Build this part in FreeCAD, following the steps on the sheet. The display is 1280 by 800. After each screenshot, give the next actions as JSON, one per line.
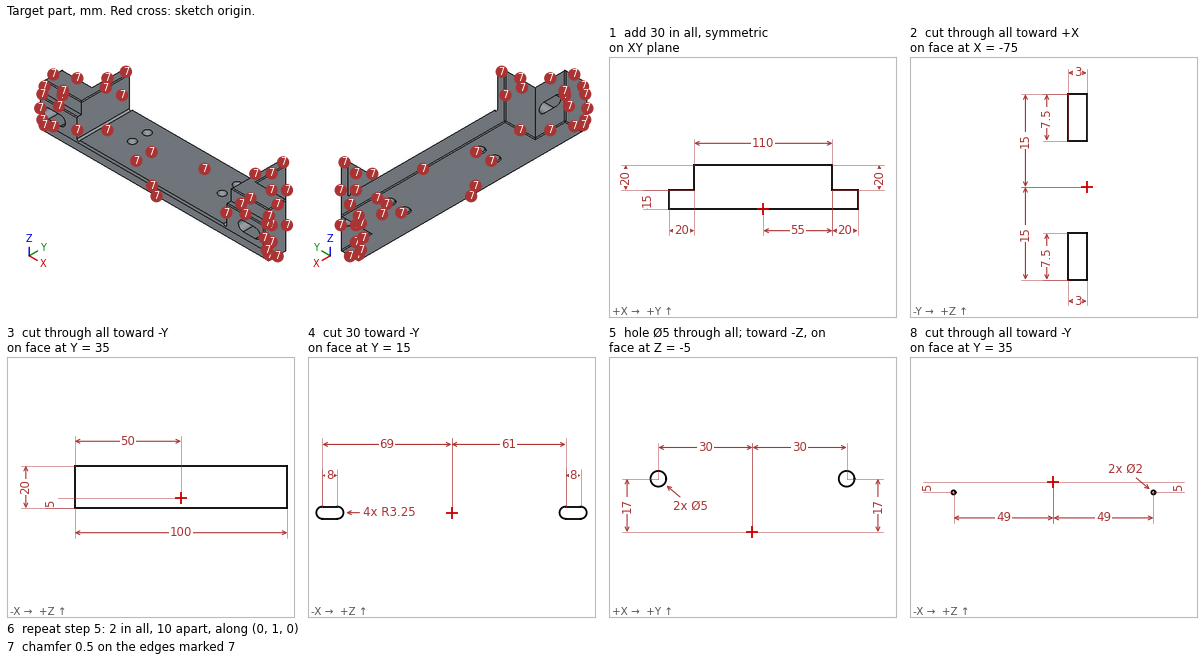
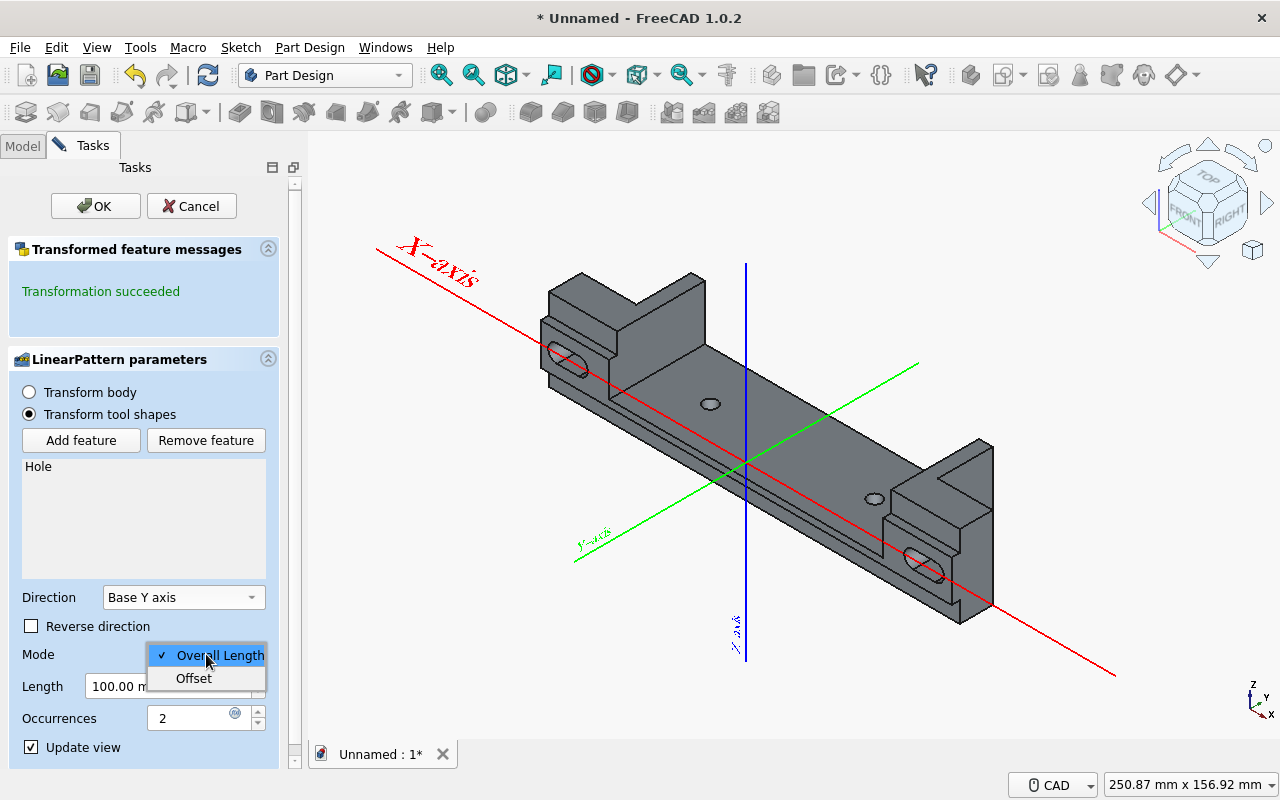
{"action": "left_click", "coordinate": [206, 678]}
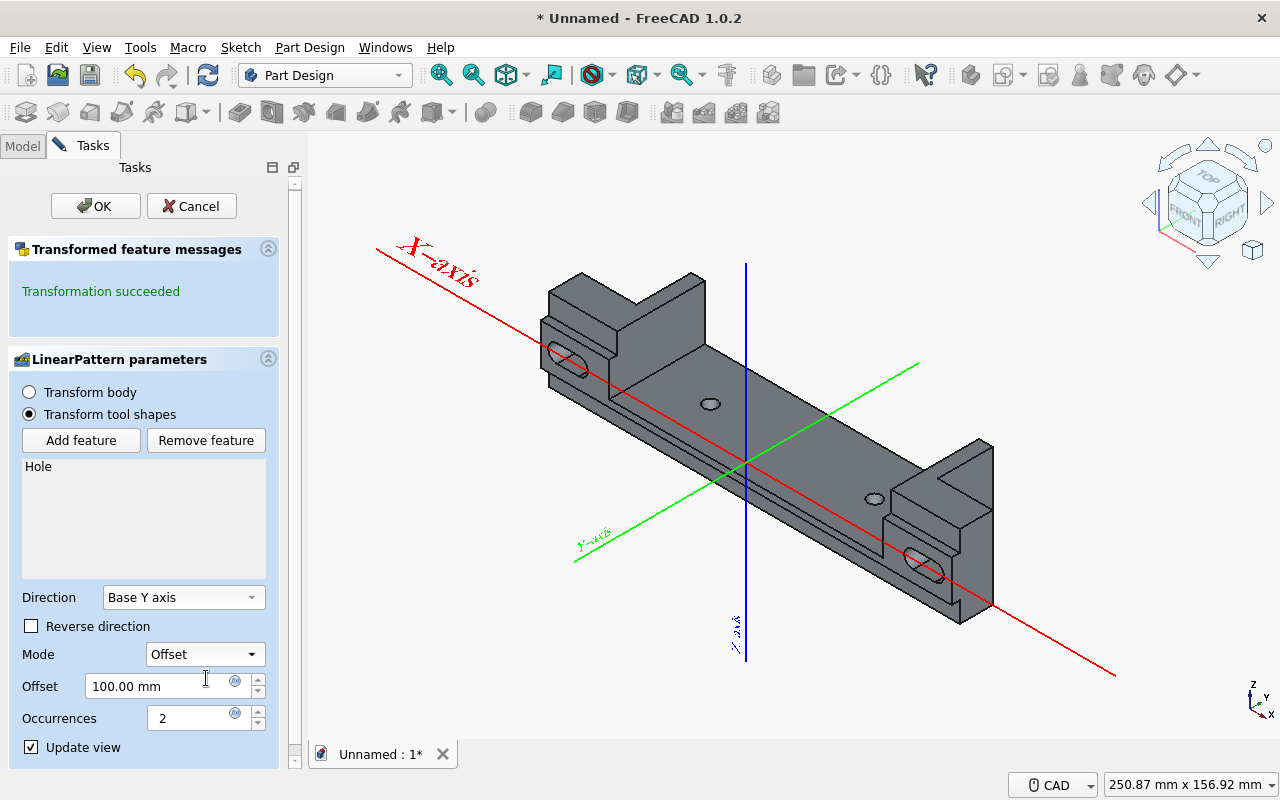
{"action": "triple_click", "coordinate": [168, 686]}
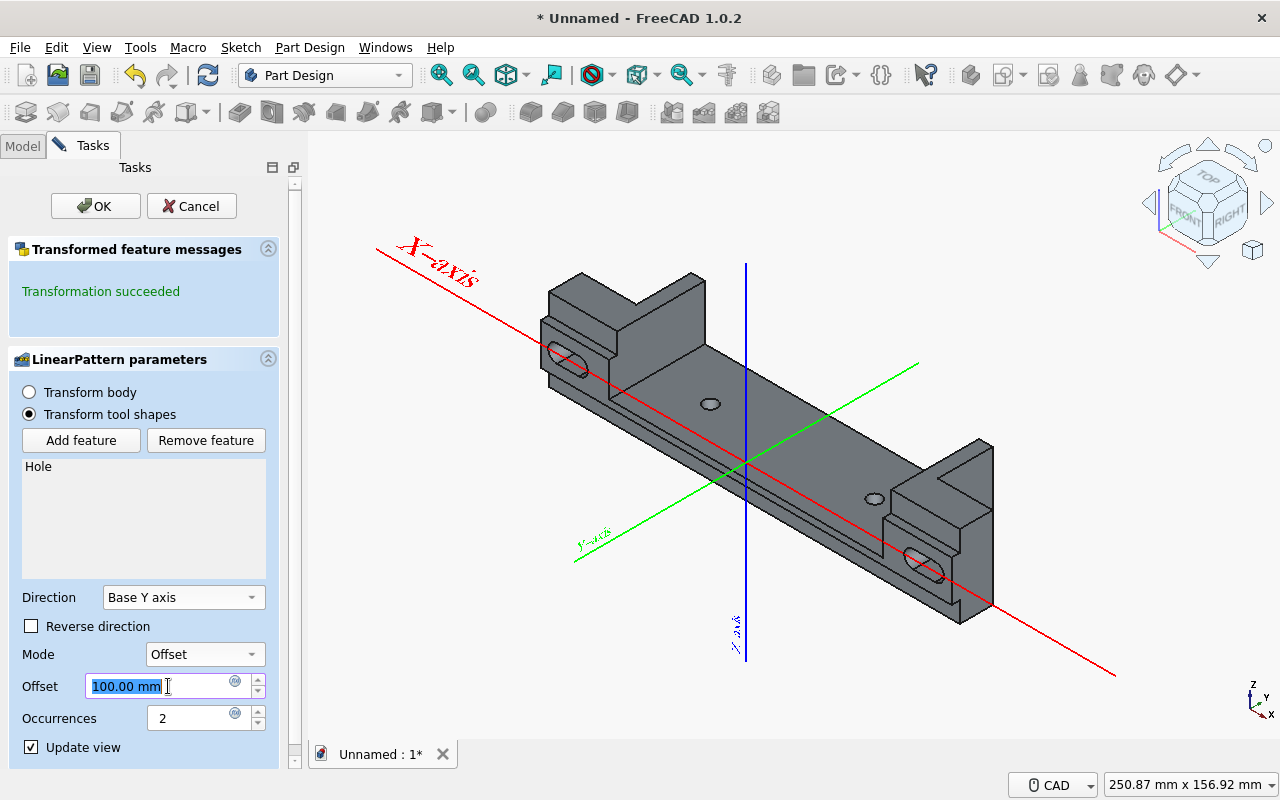
{"action": "type", "text": "10"}
{"action": "key", "text": "Tab"}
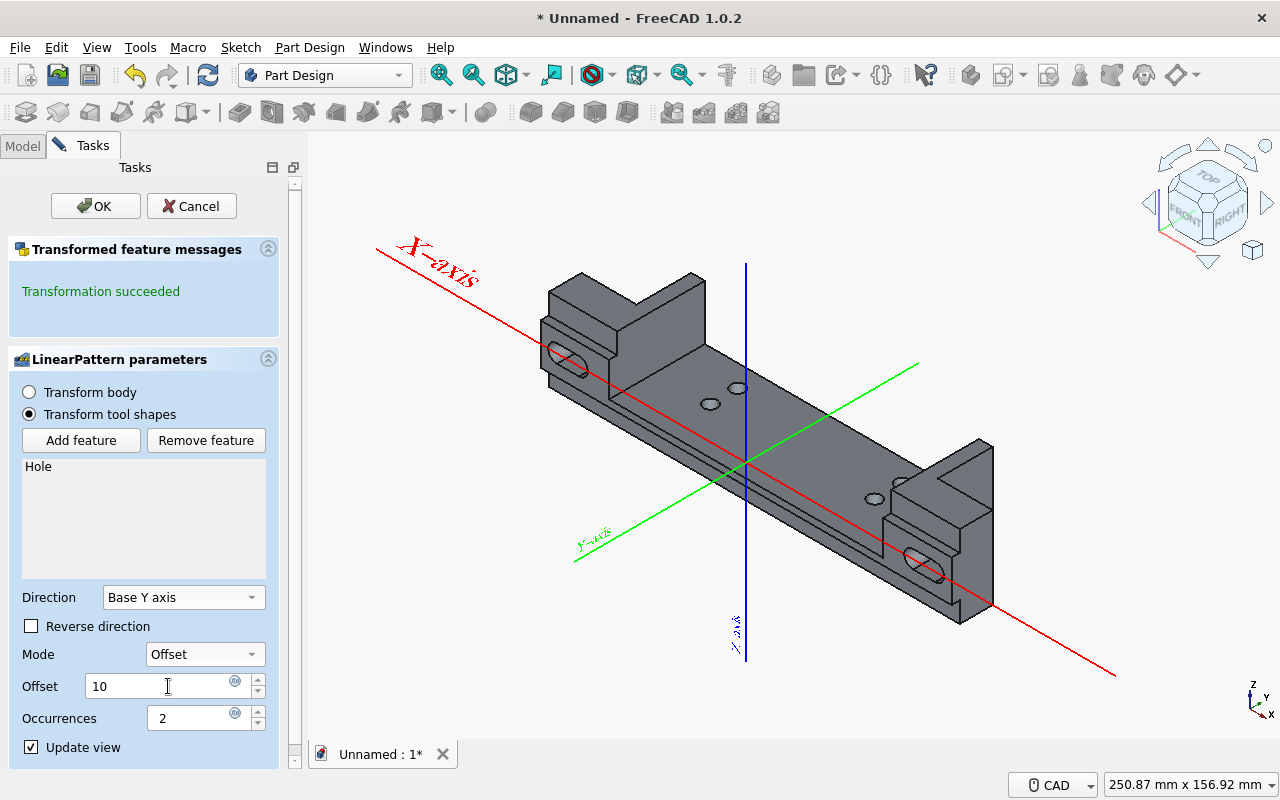
{"action": "triple_click", "coordinate": [198, 718]}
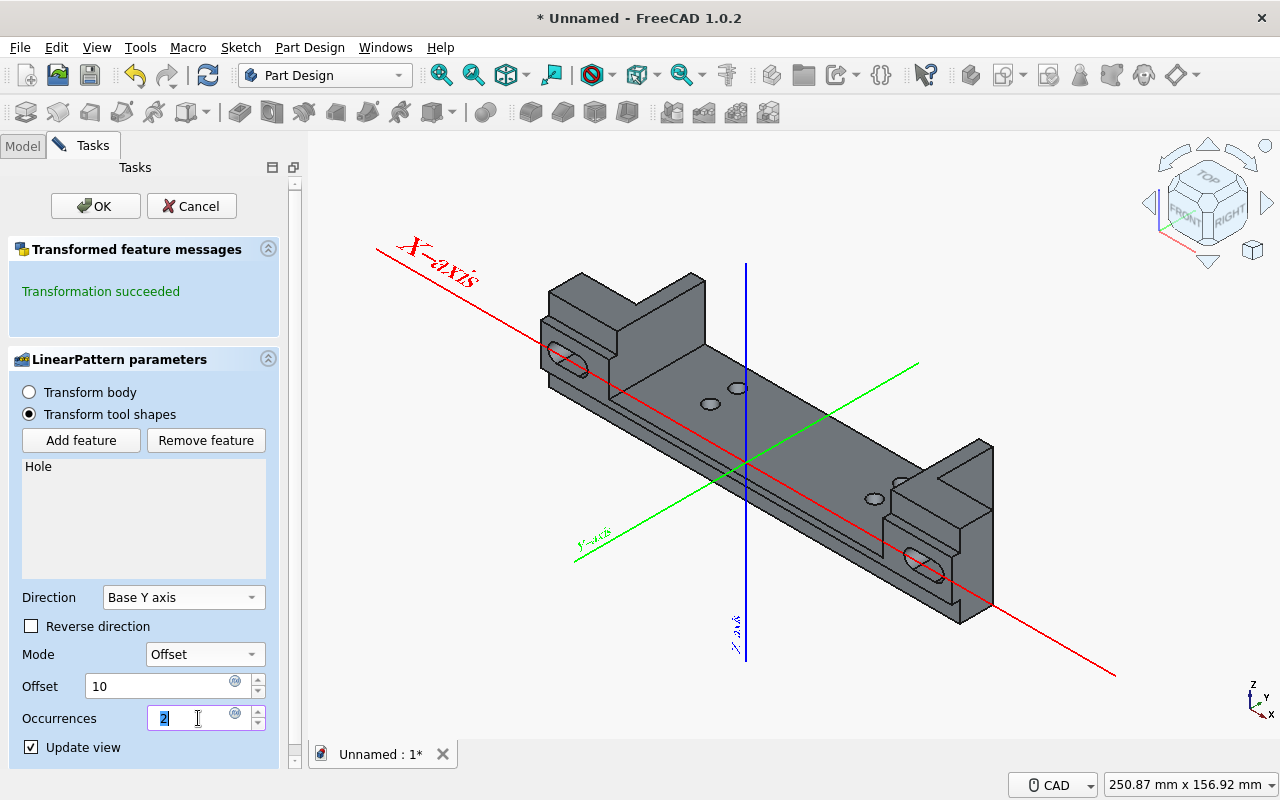
{"action": "type", "text": "2"}
{"action": "key", "text": "Tab"}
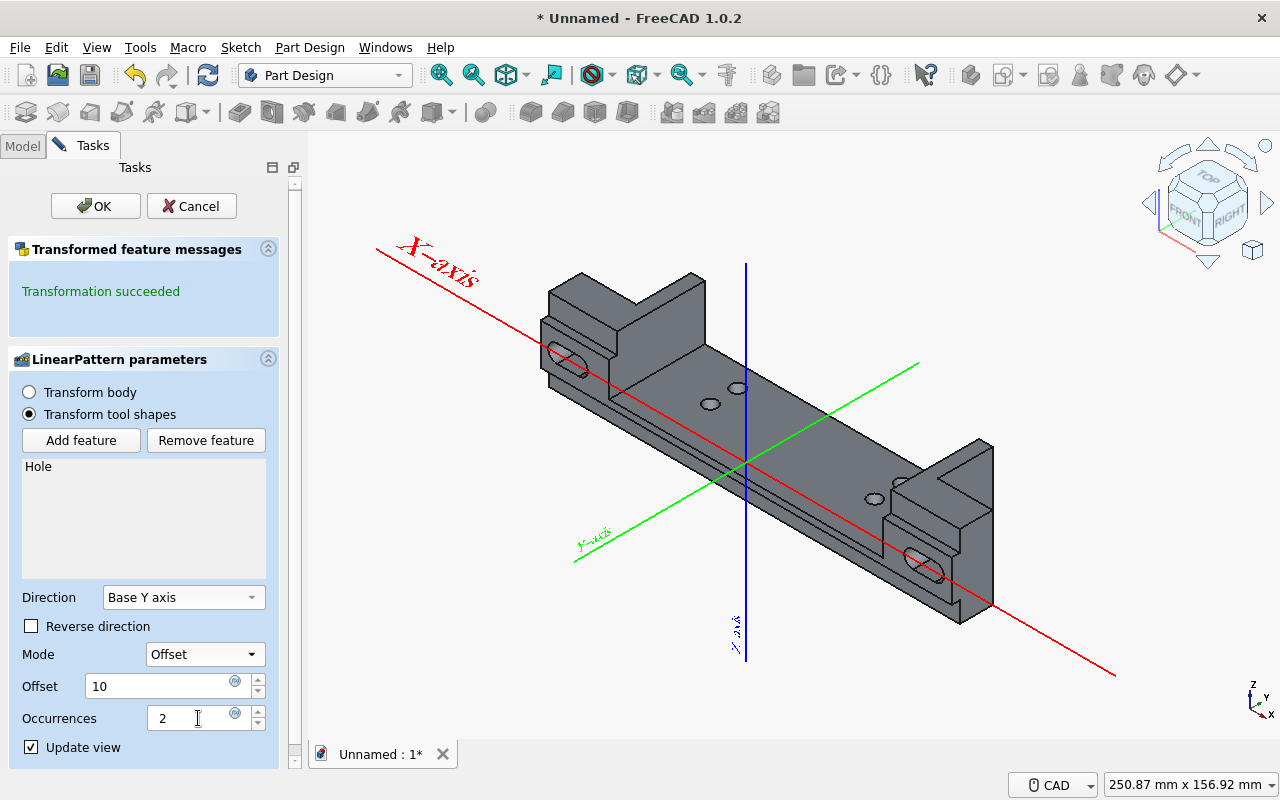
{"action": "left_click", "coordinate": [96, 206]}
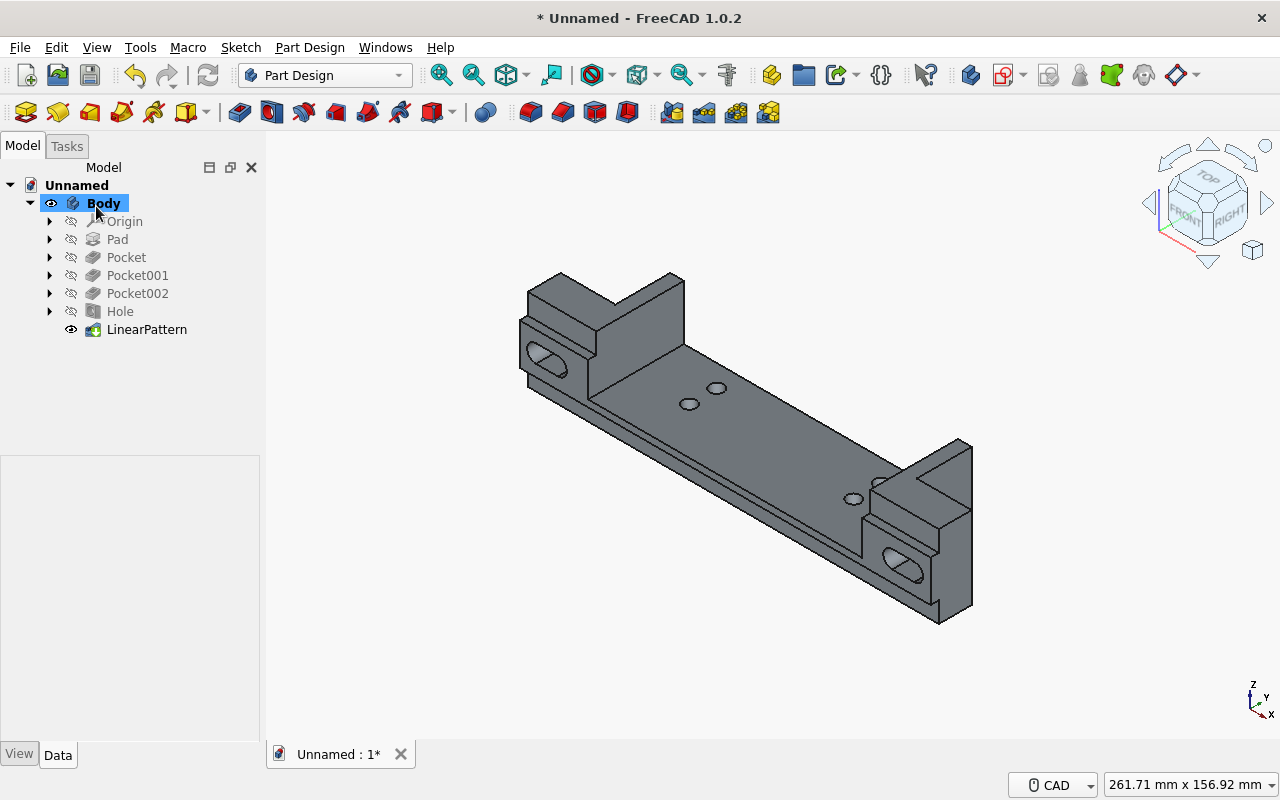
{"action": "left_click", "coordinate": [951, 568]}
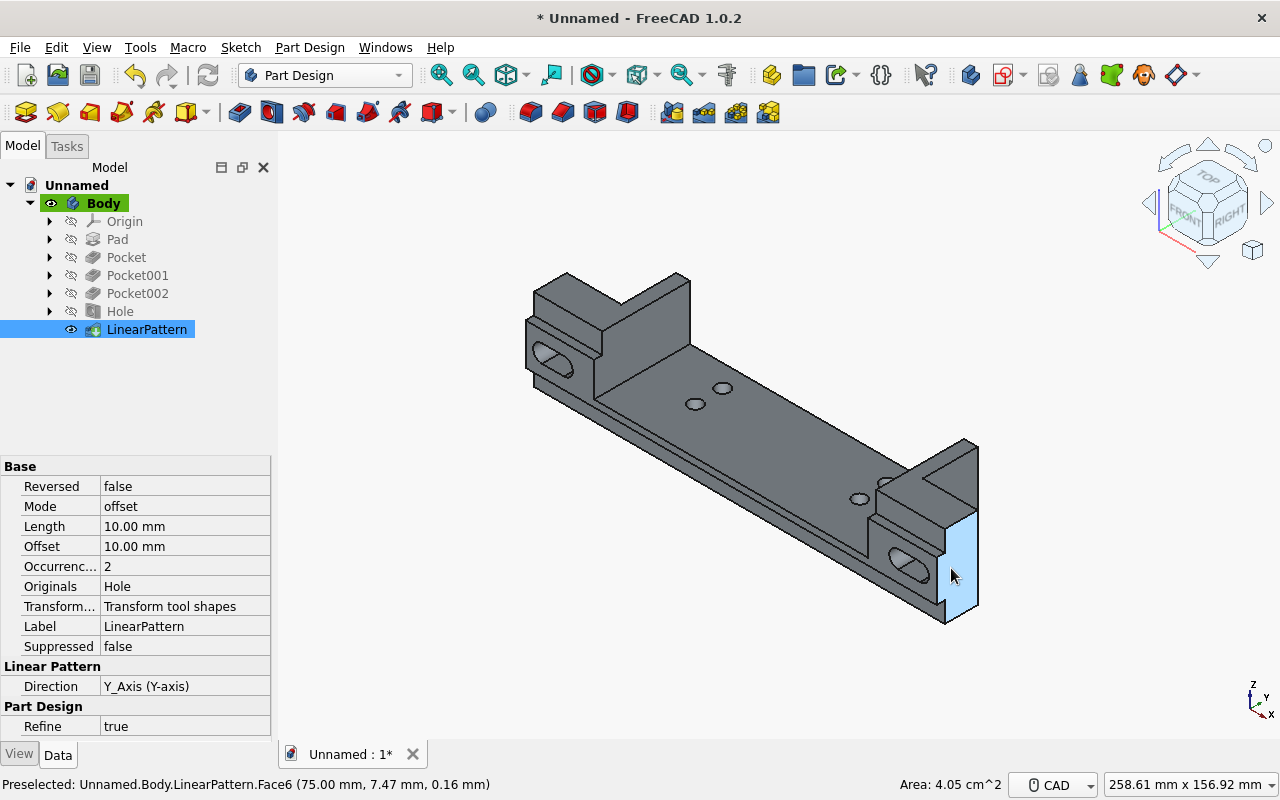
{"action": "left_click", "coordinate": [606, 311], "text": "ctrl"}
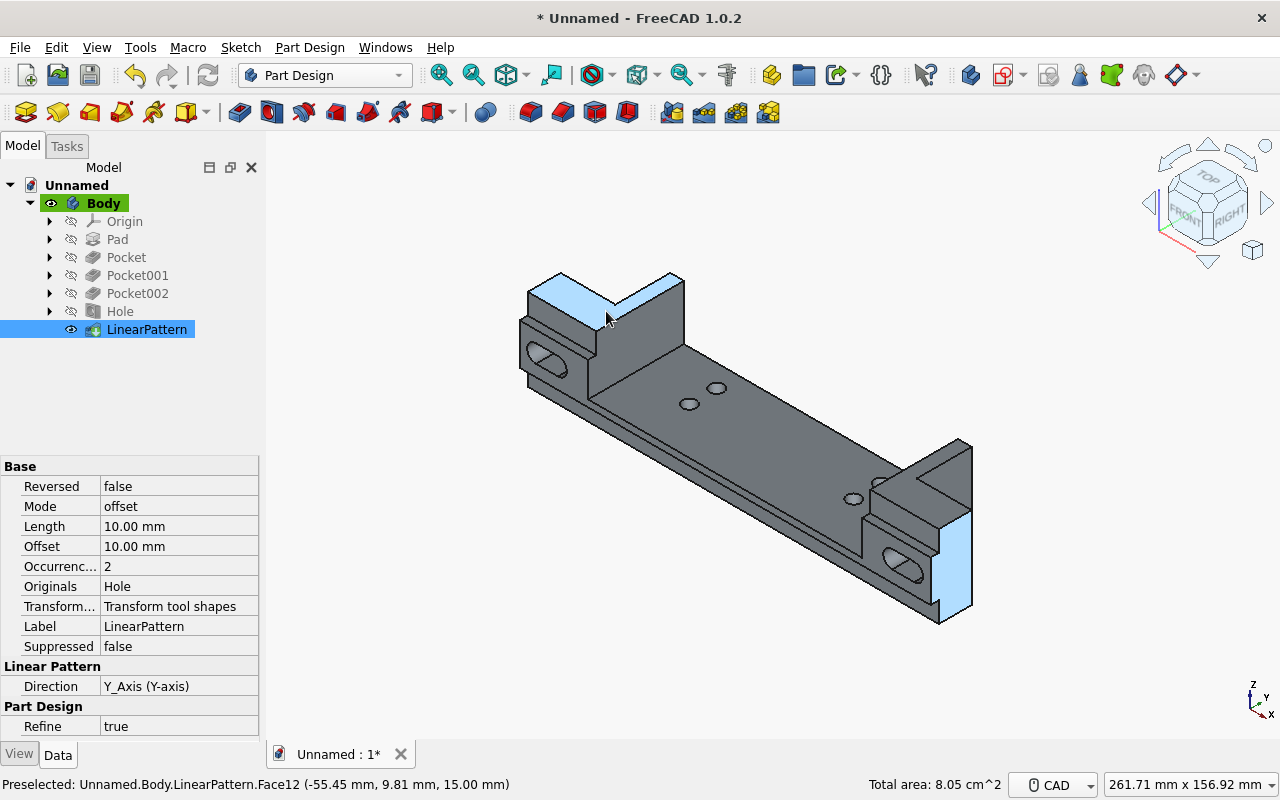
{"action": "left_click", "coordinate": [943, 509], "text": "ctrl"}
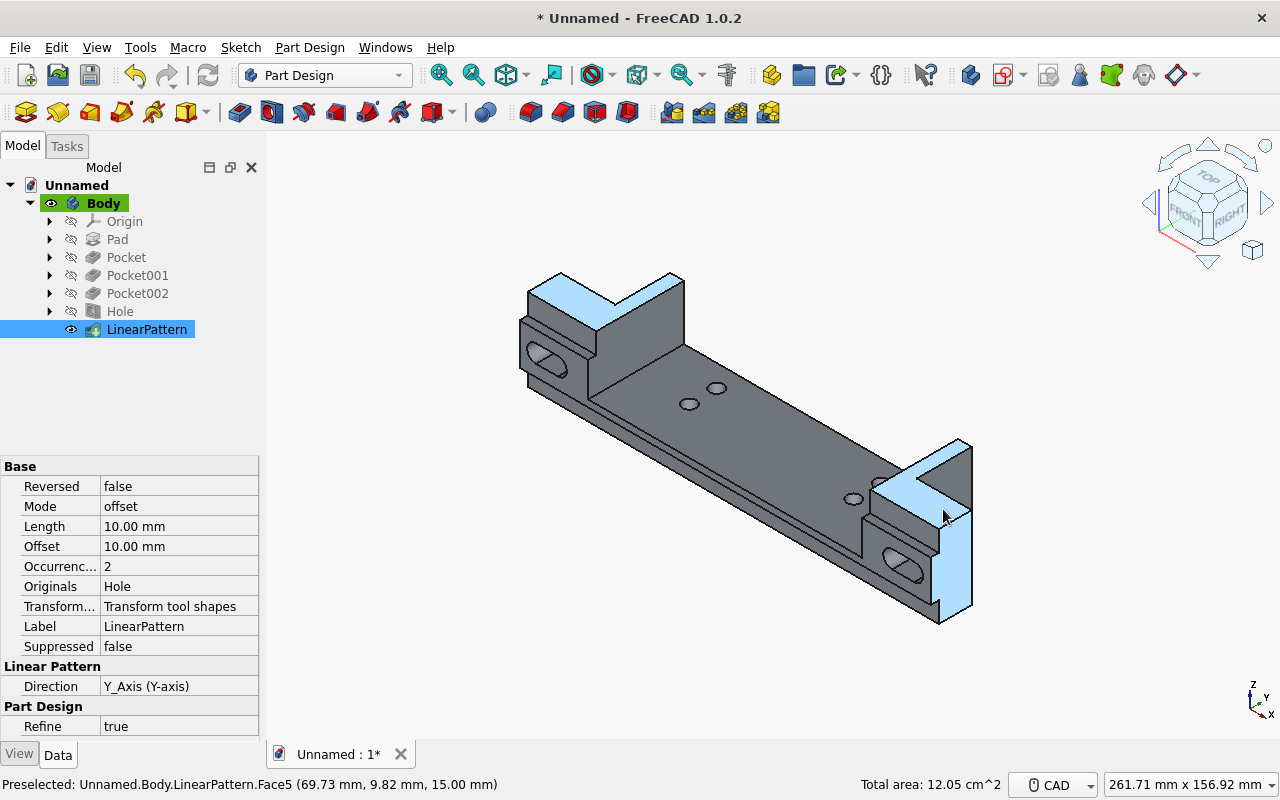
{"action": "left_click", "coordinate": [896, 537], "text": "ctrl"}